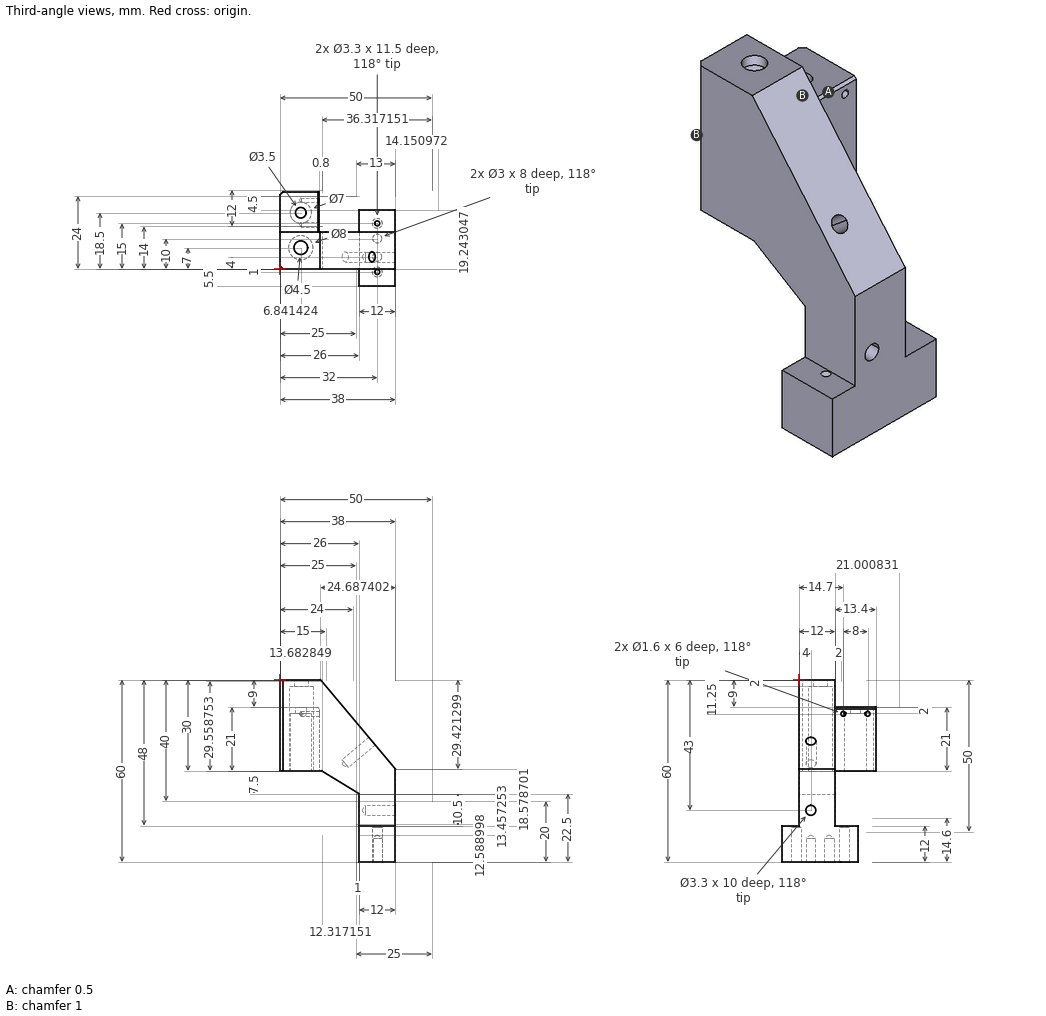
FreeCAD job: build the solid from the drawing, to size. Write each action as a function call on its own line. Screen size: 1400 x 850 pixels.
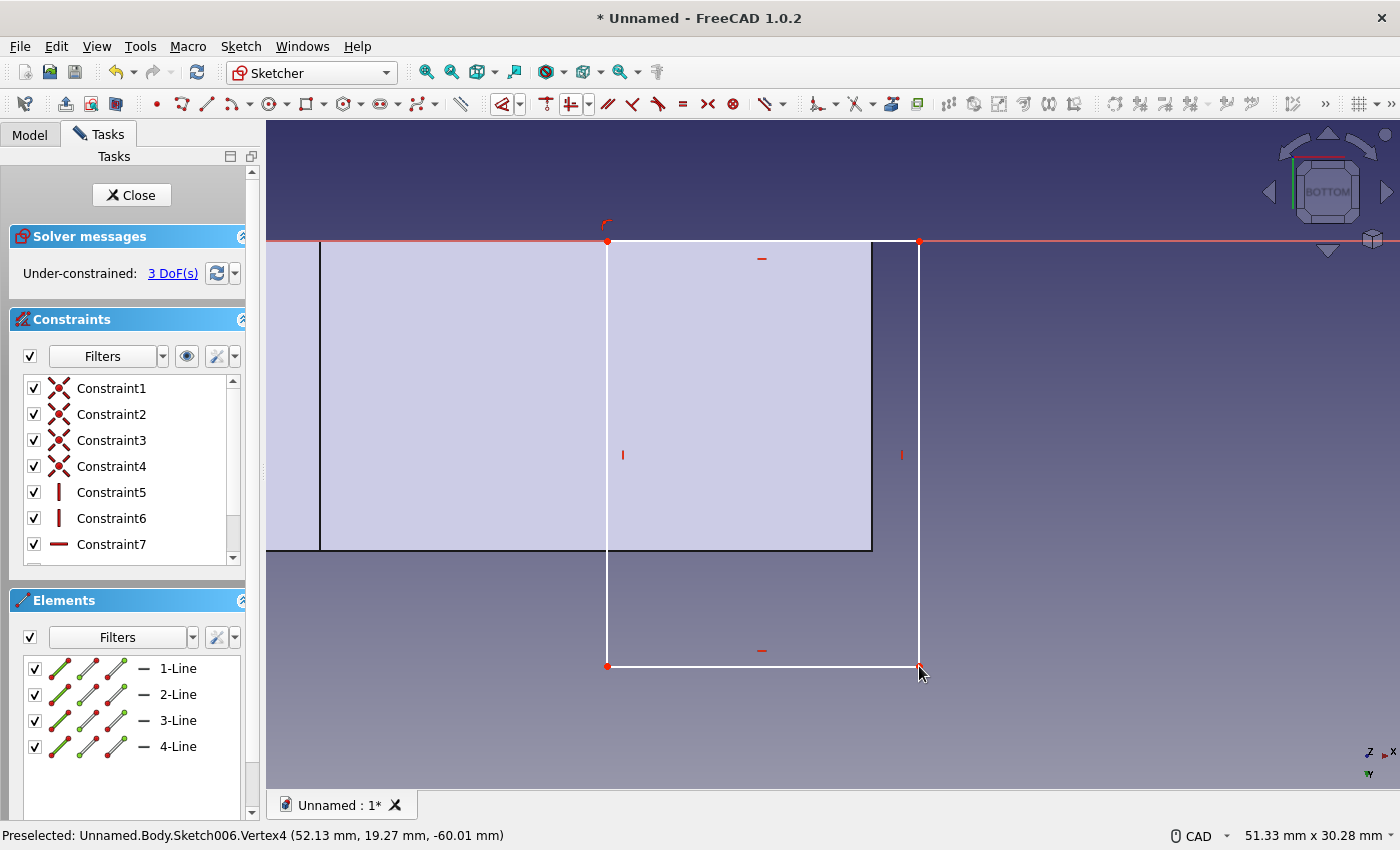
click(607, 241)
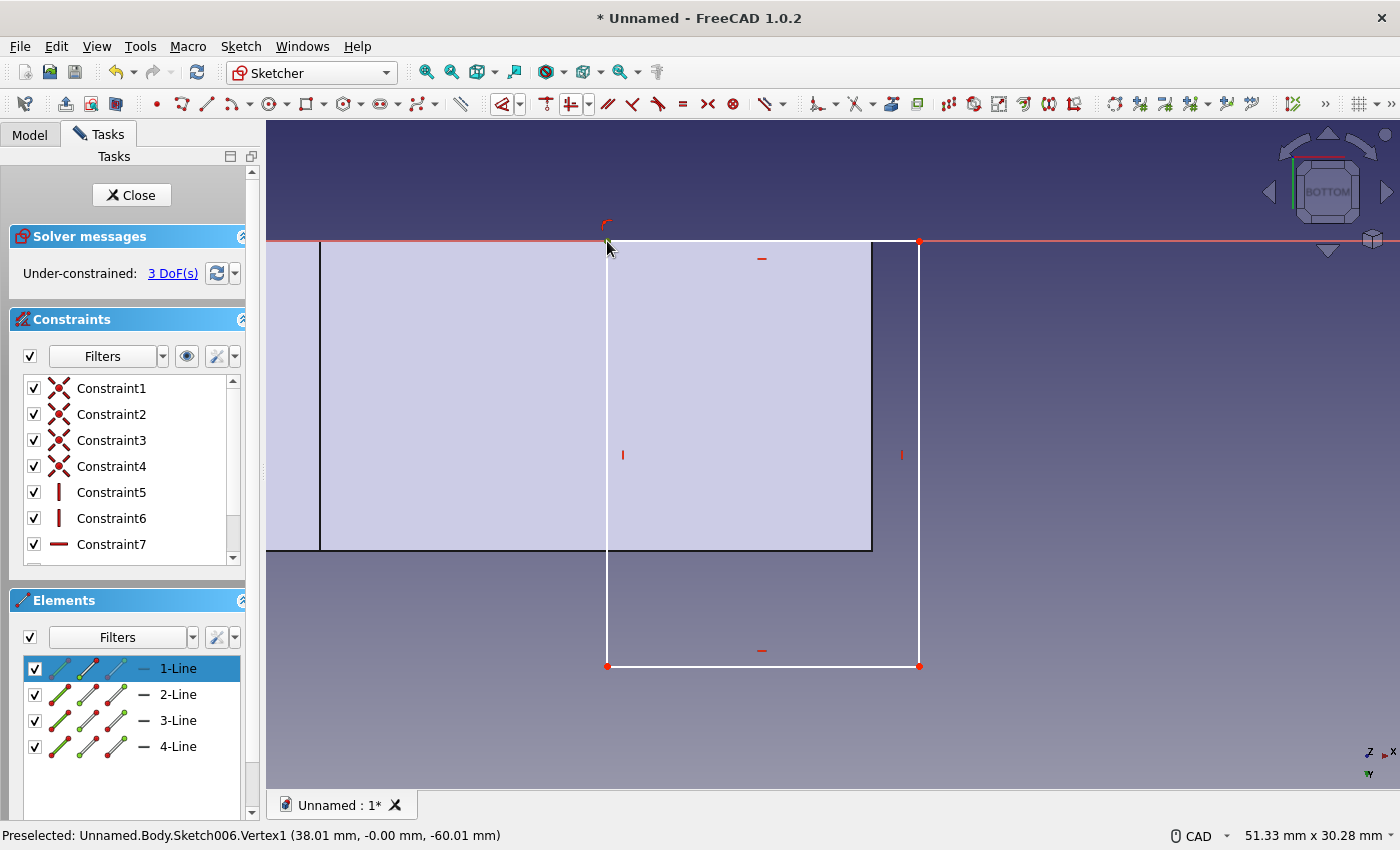
click(520, 104)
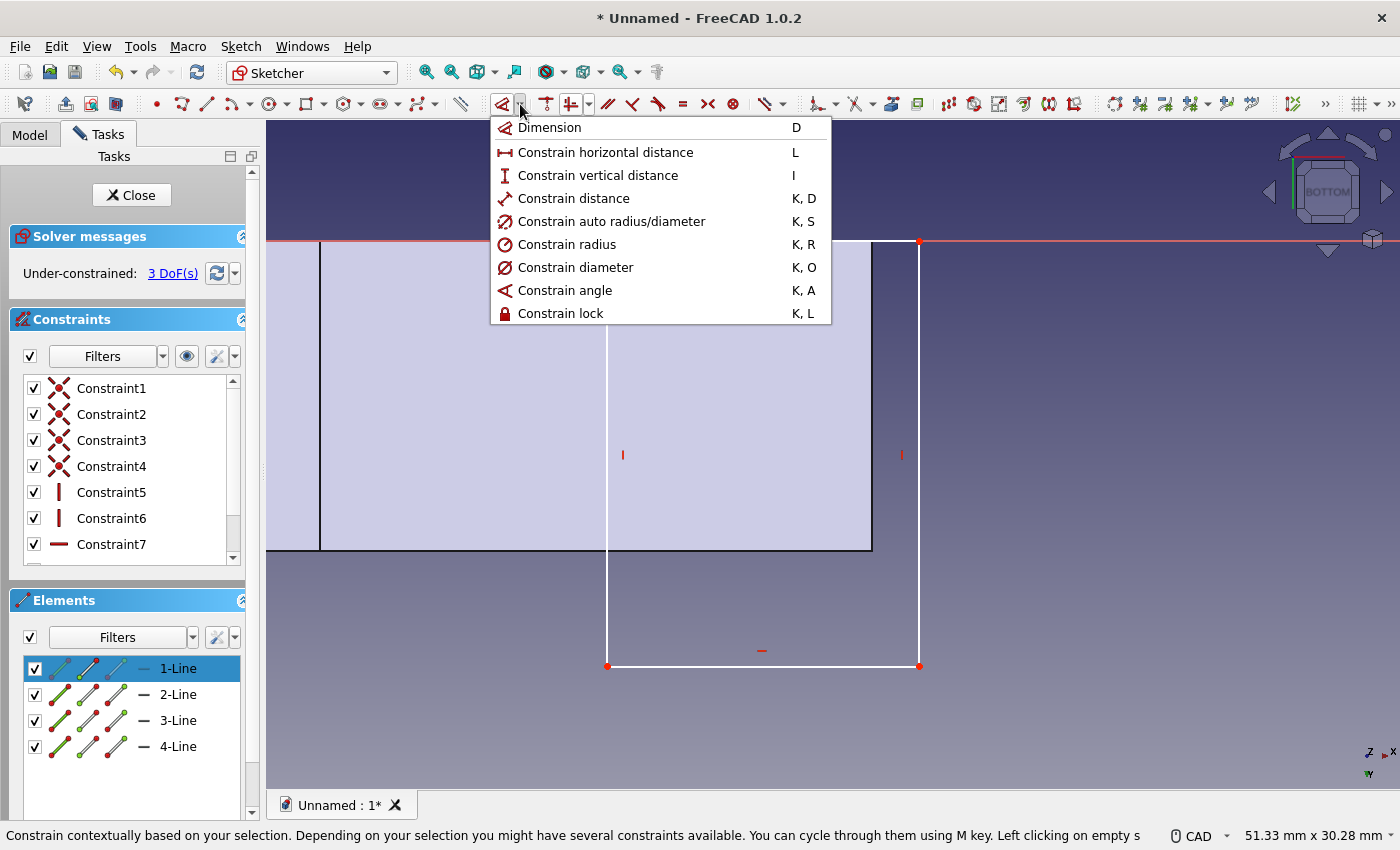
click(661, 152)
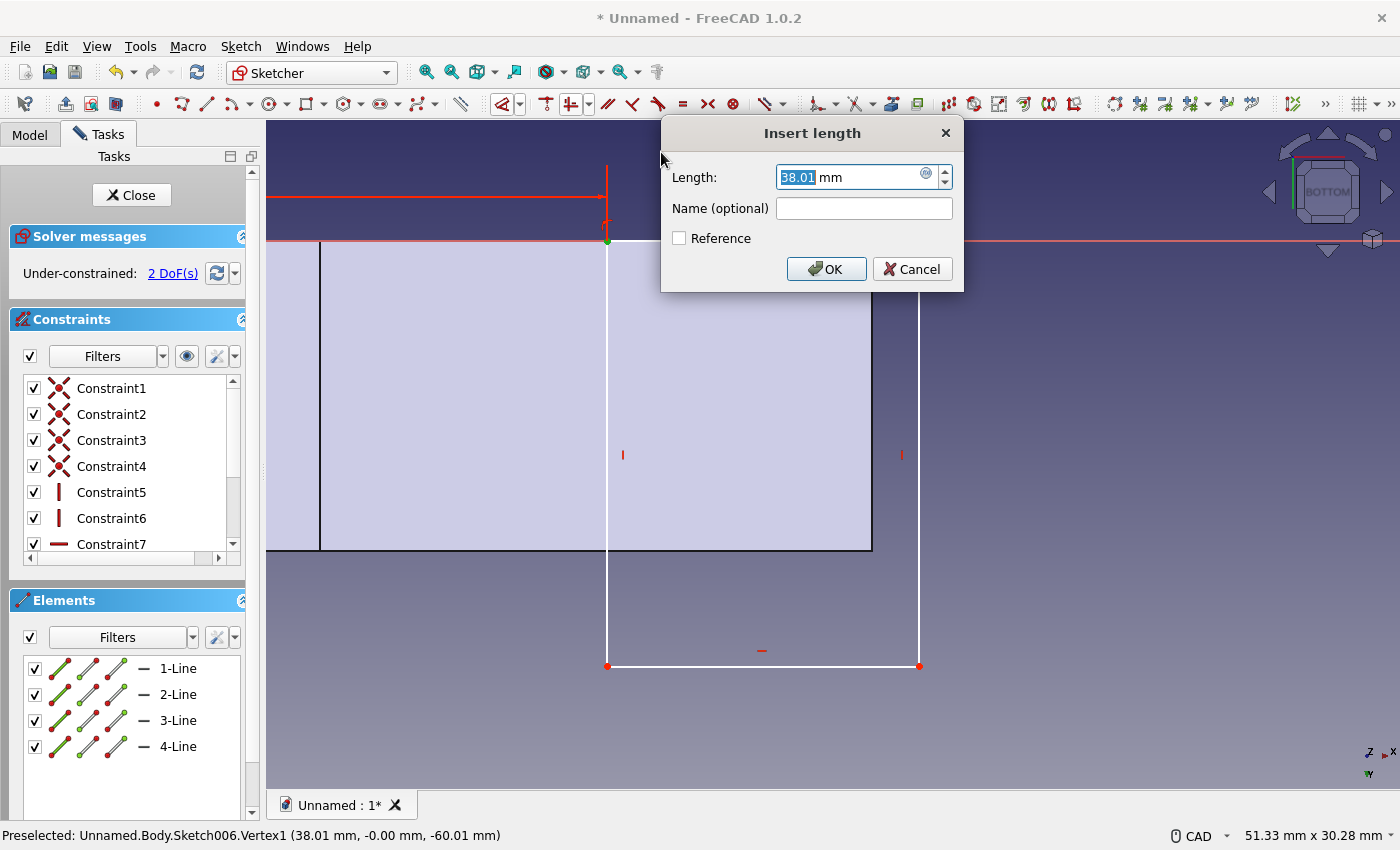
text(38)
key(Return)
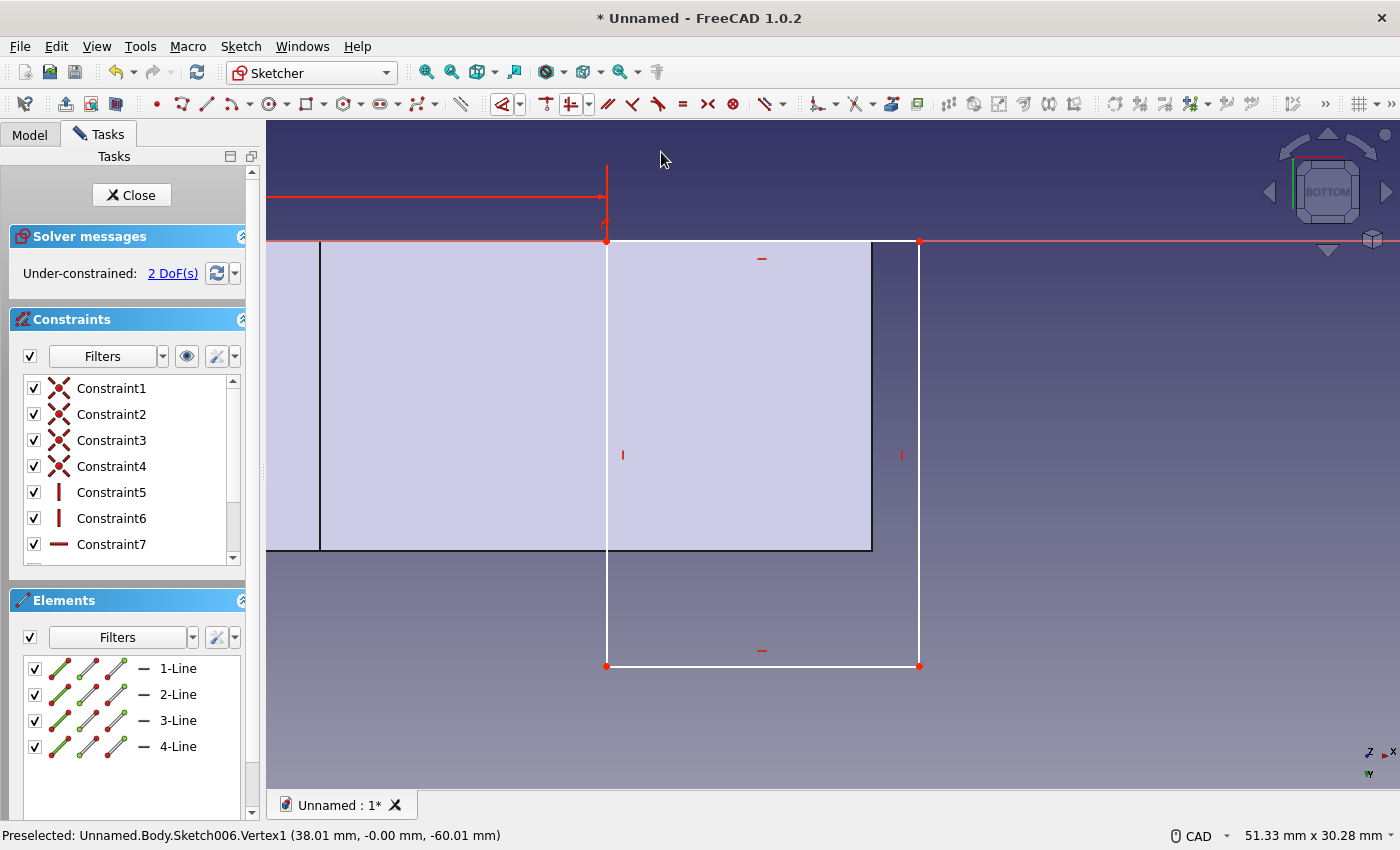
click(607, 369)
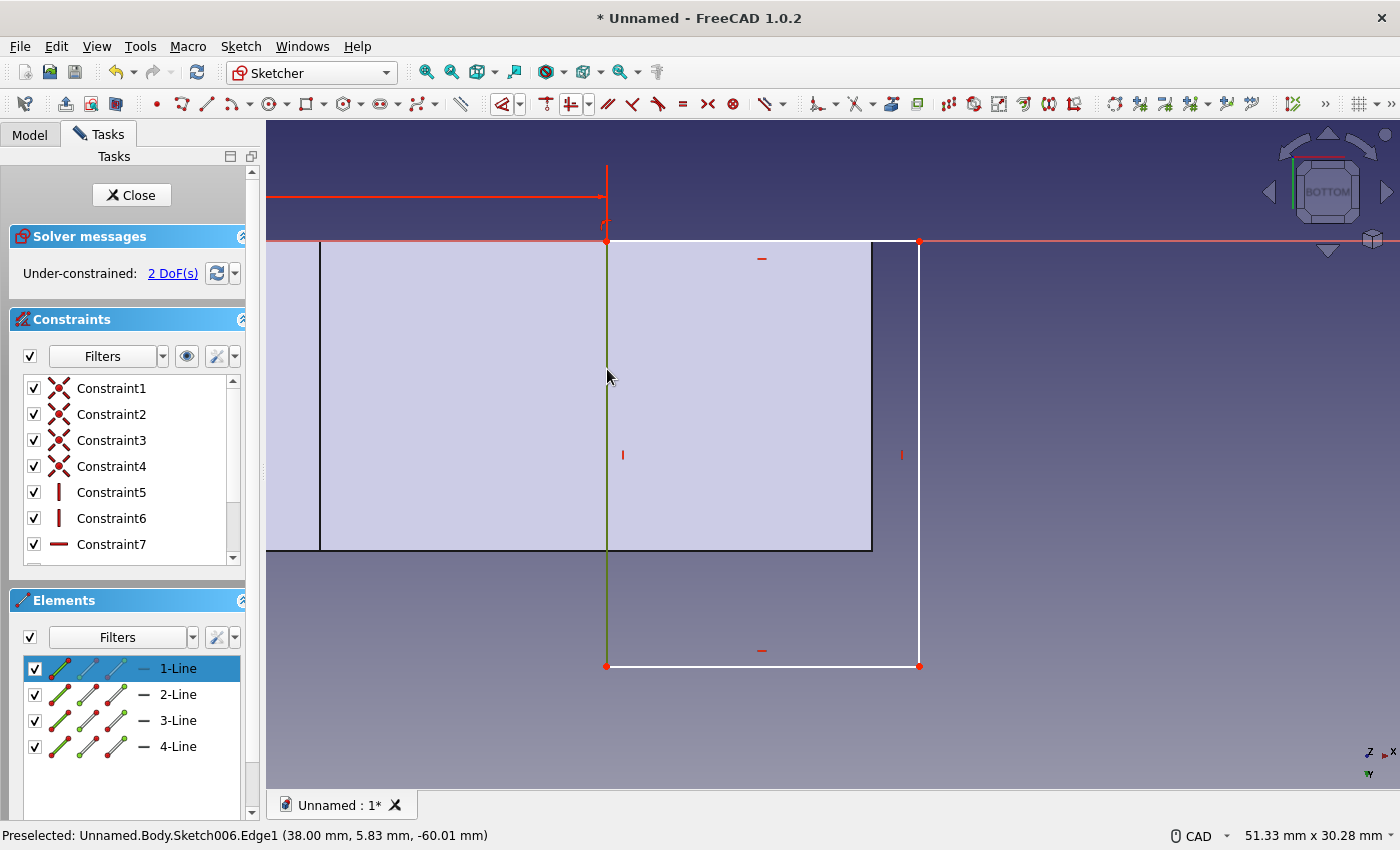
click(520, 104)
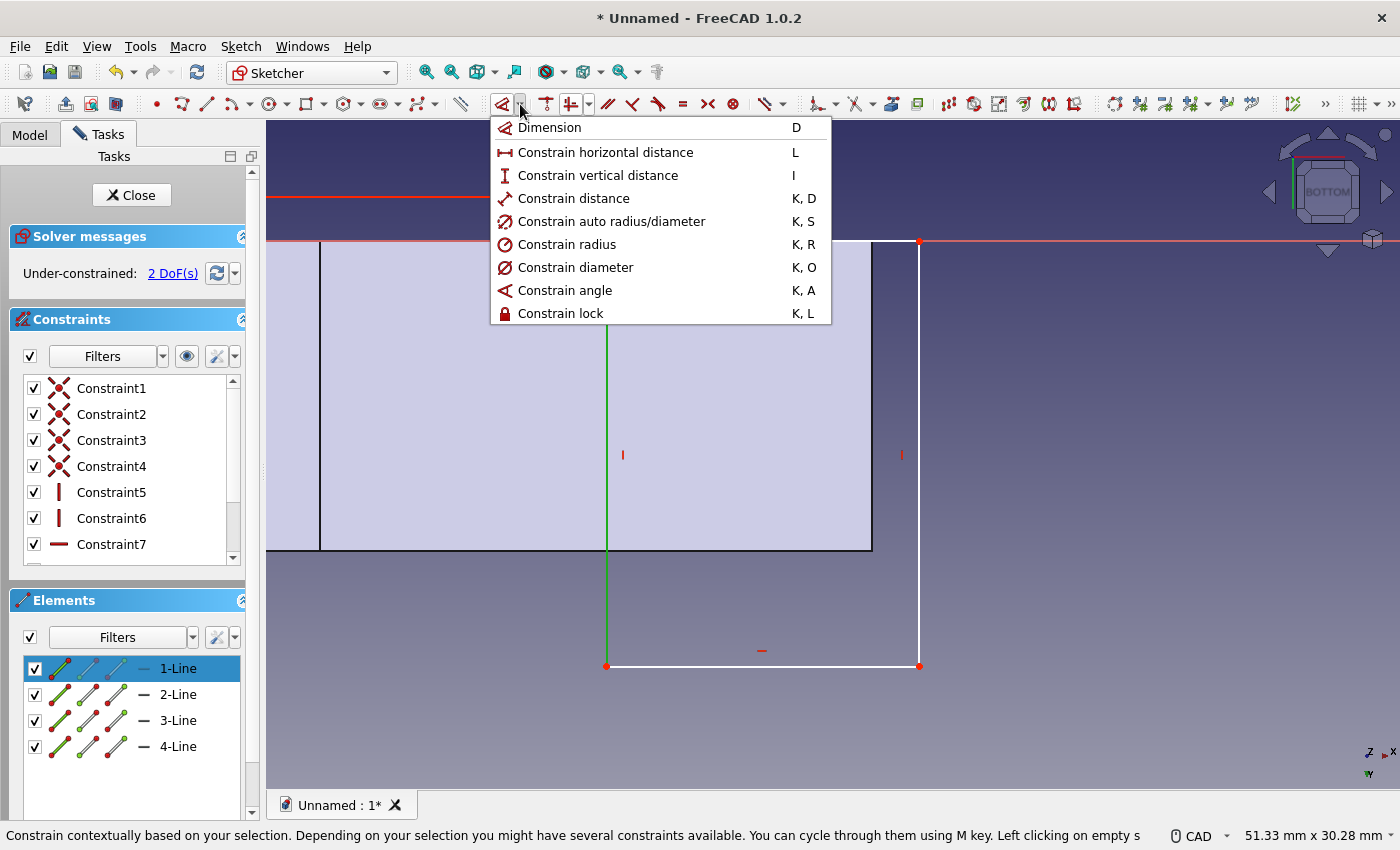
click(661, 176)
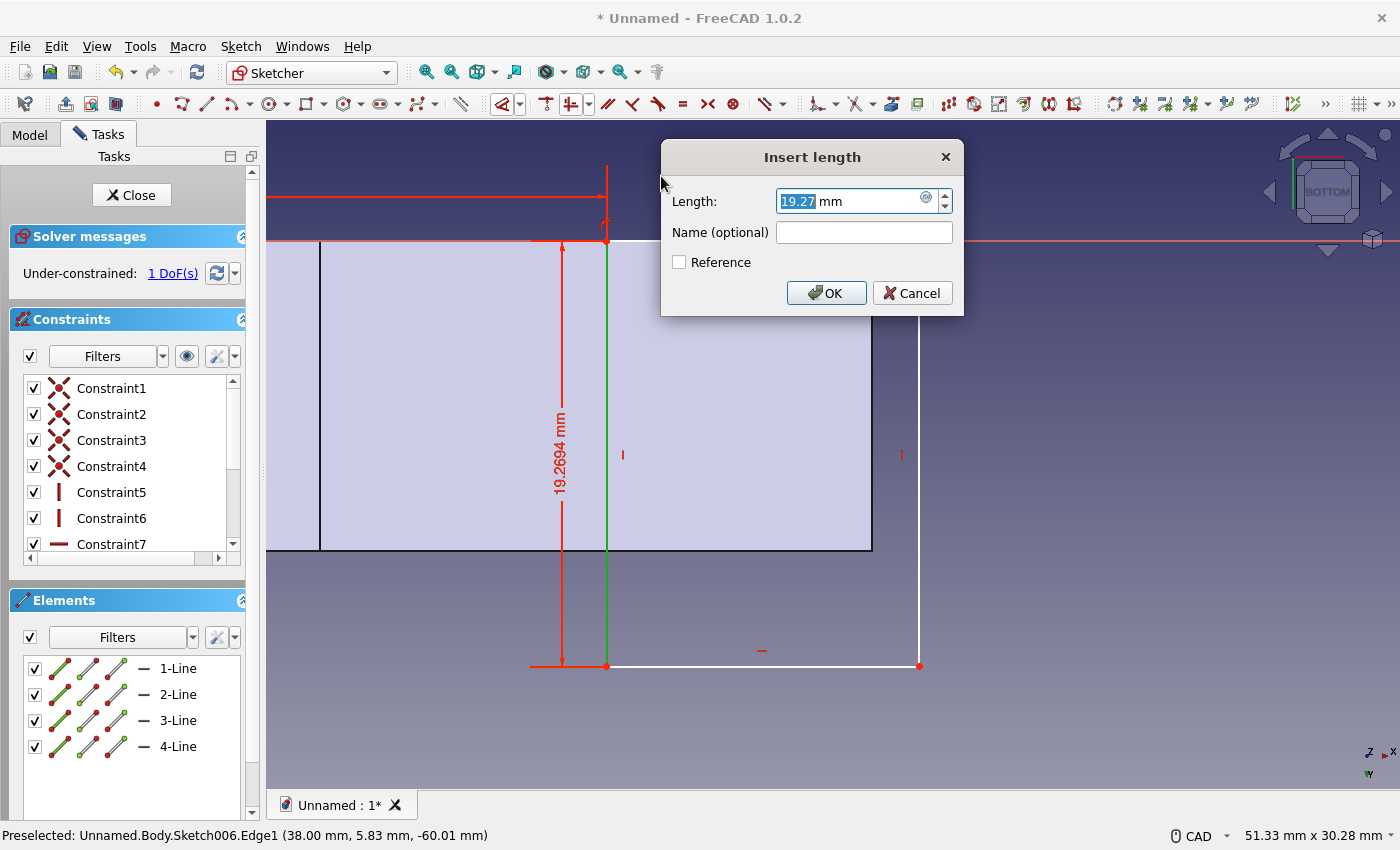
text(19.243047)
key(Return)